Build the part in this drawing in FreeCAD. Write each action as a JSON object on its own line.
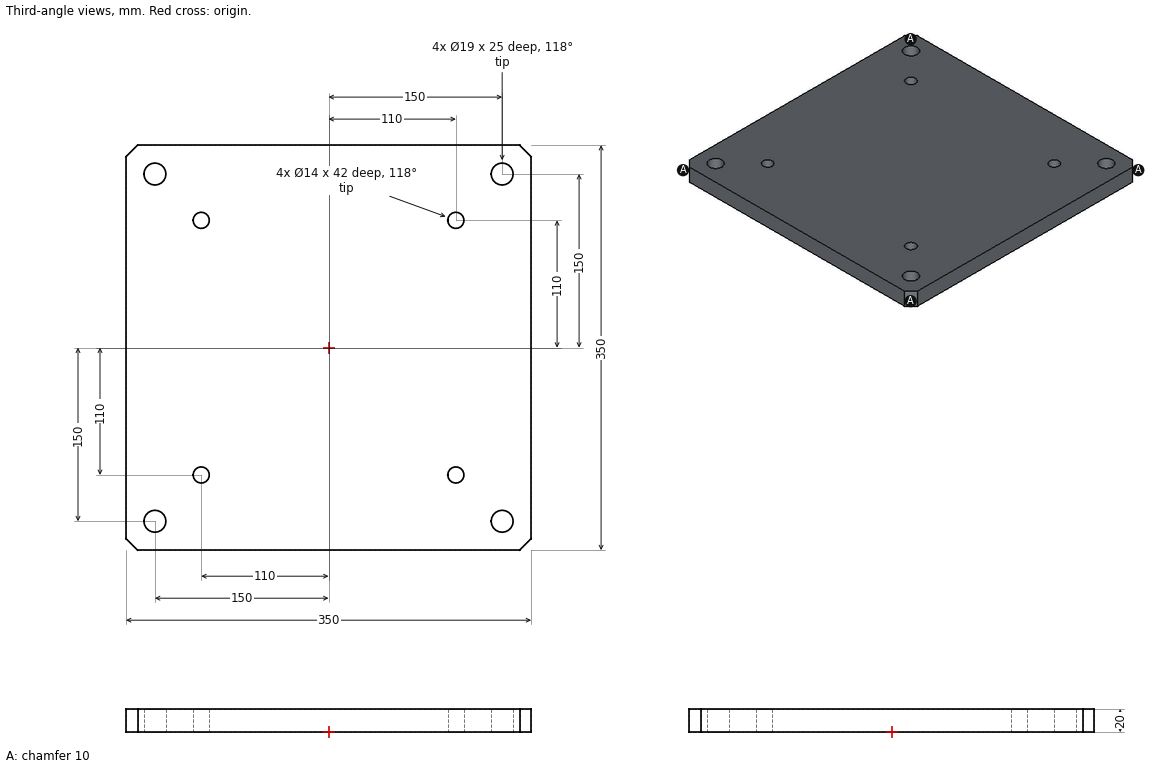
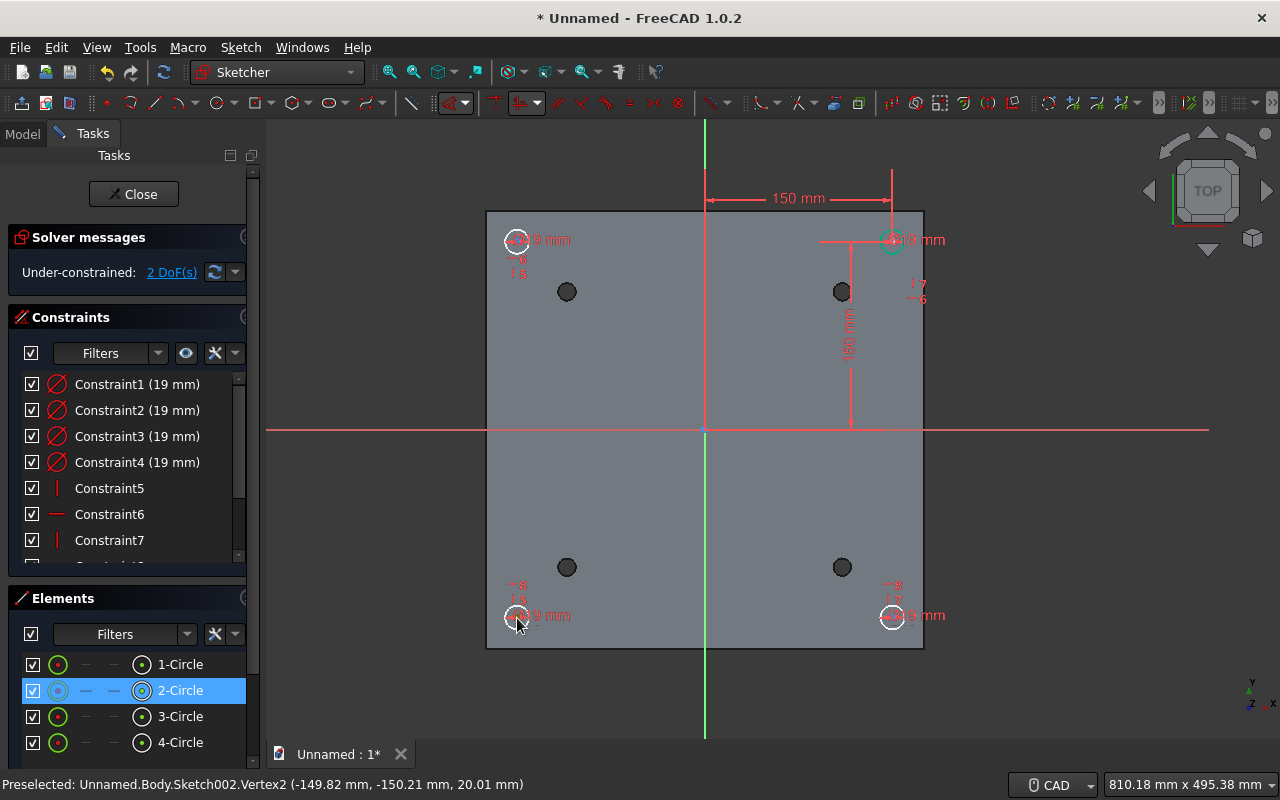
{"action": "key", "text": "l"}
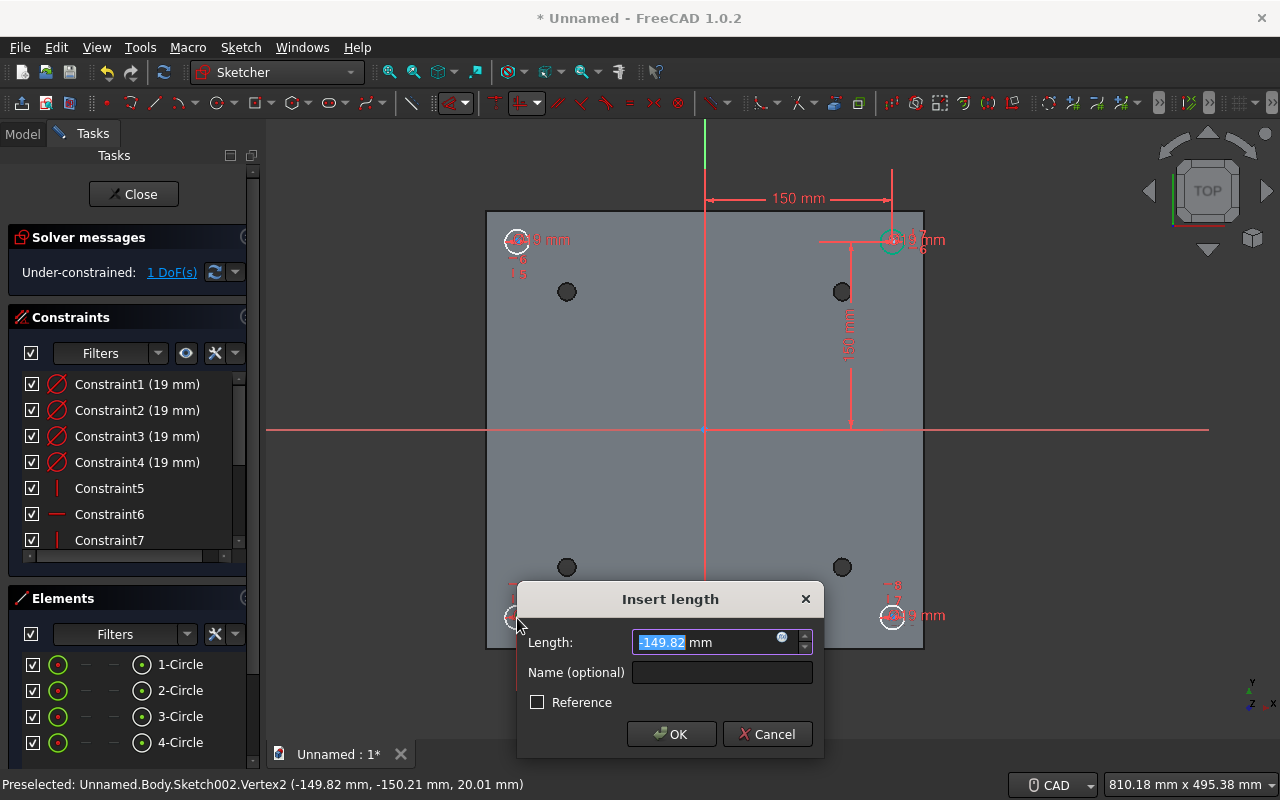
{"action": "type", "text": "-150"}
{"action": "key", "text": "Return"}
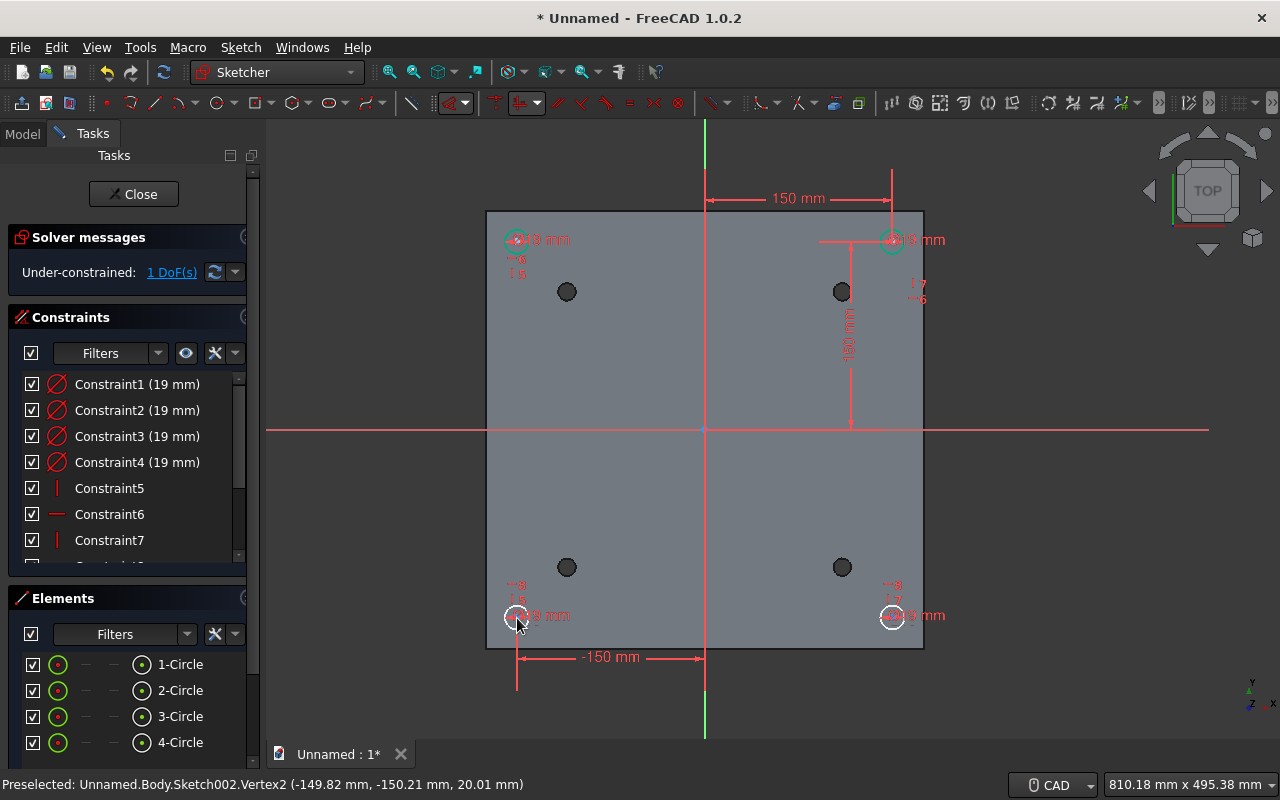
{"action": "left_click", "coordinate": [517, 618]}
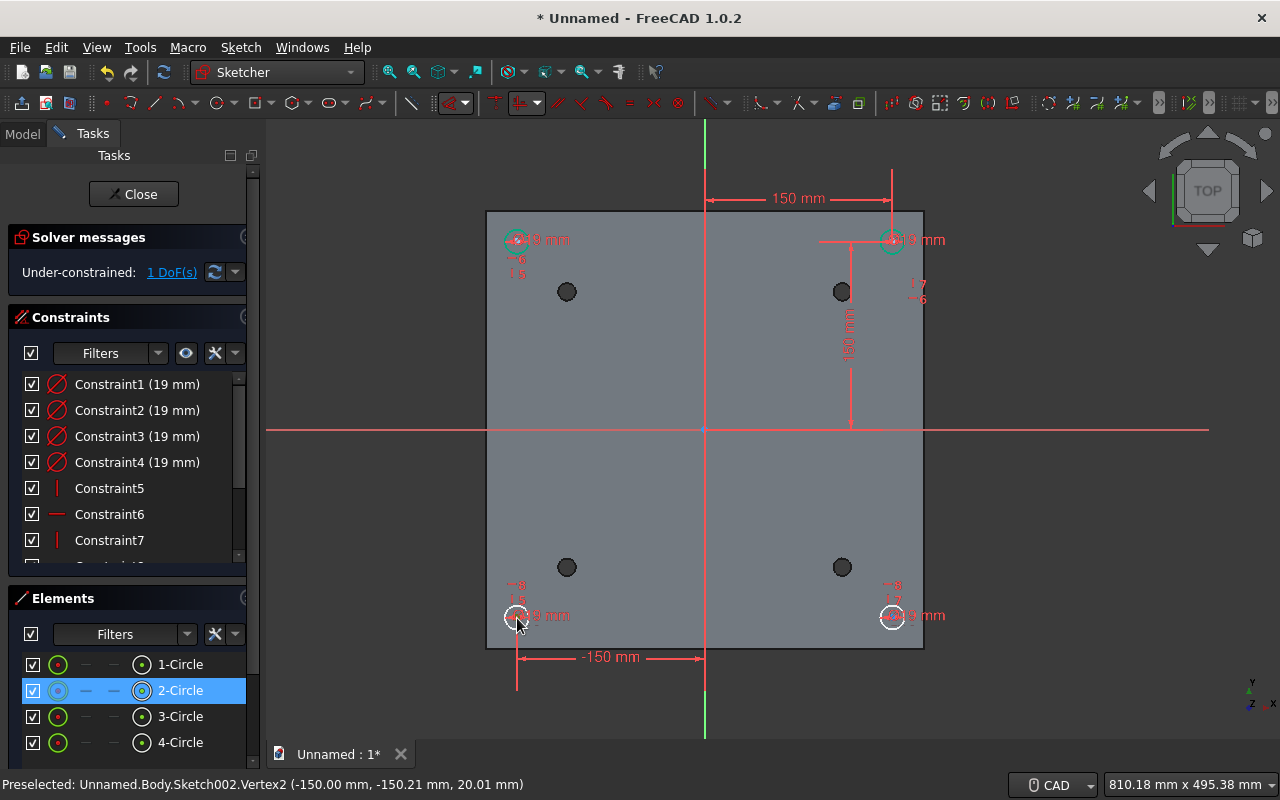
{"action": "key", "text": "i"}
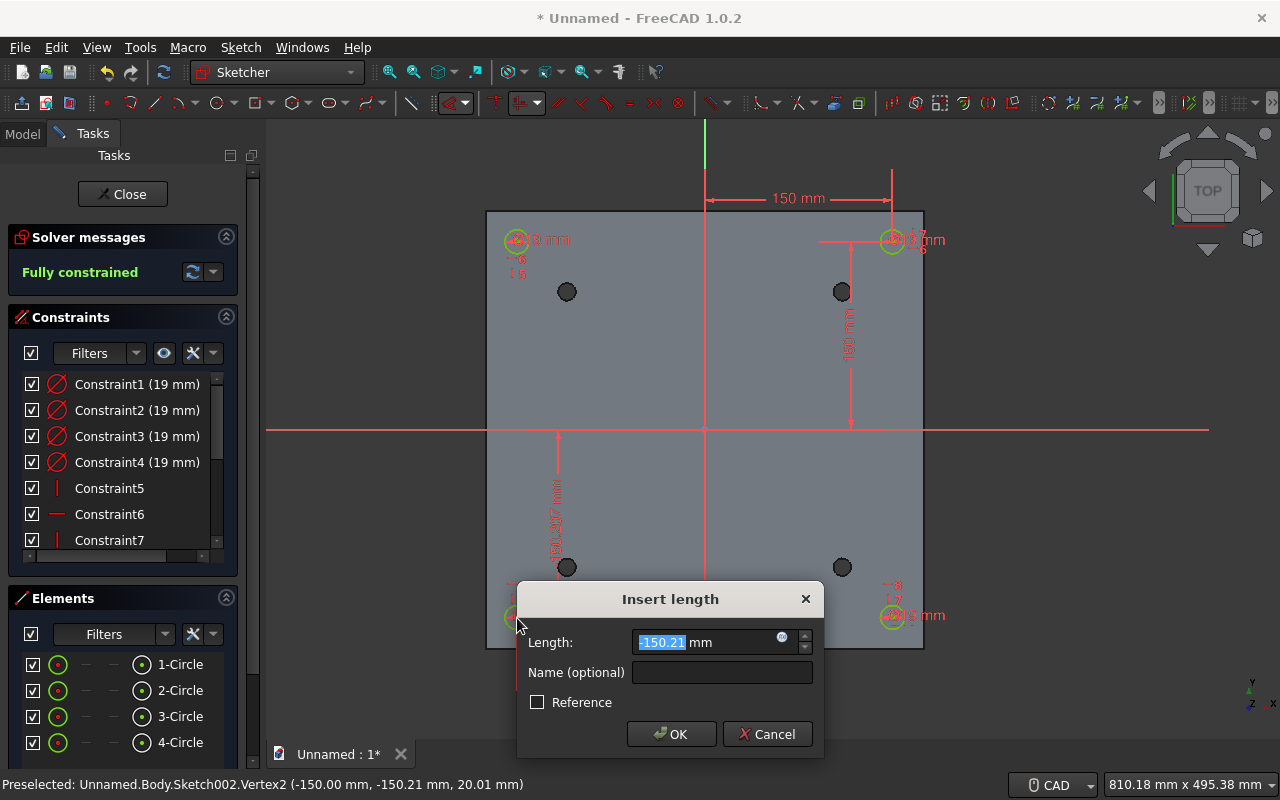
{"action": "type", "text": "-150"}
{"action": "key", "text": "Return"}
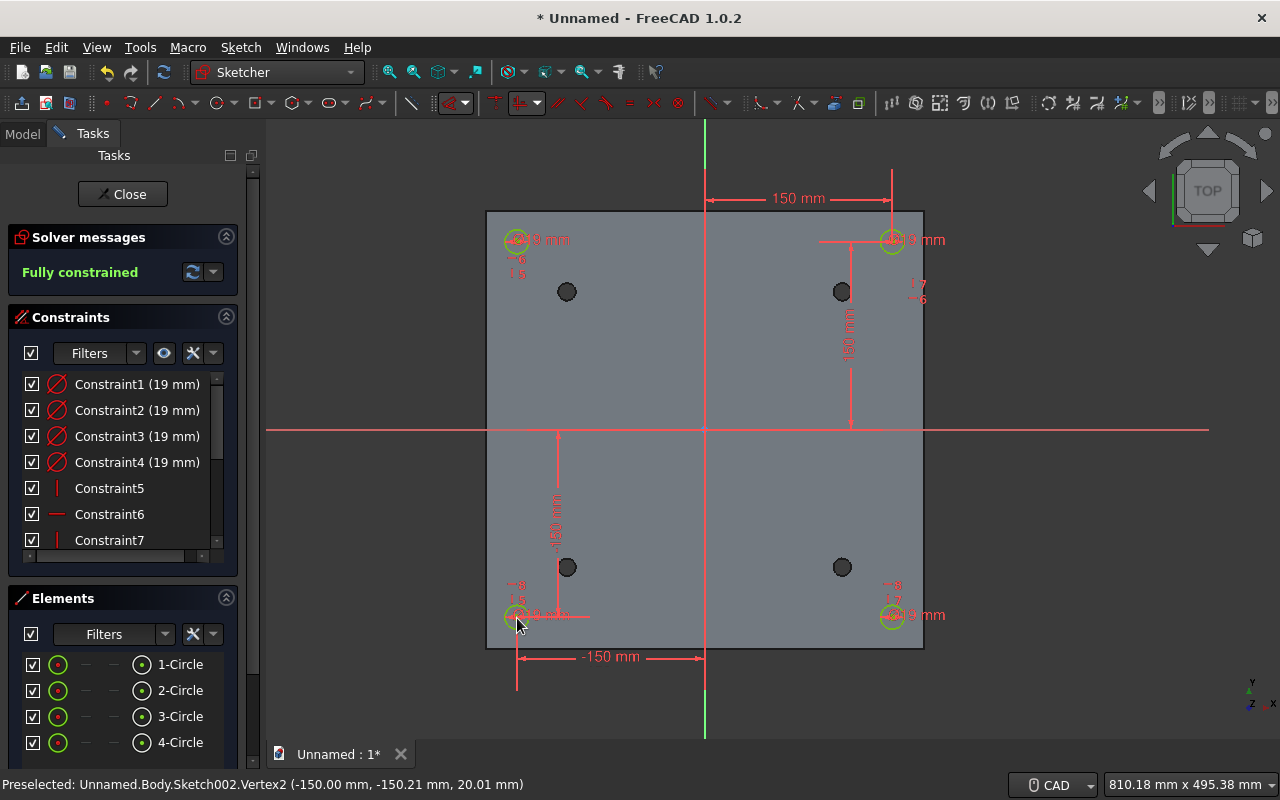
{"action": "left_click", "coordinate": [123, 194]}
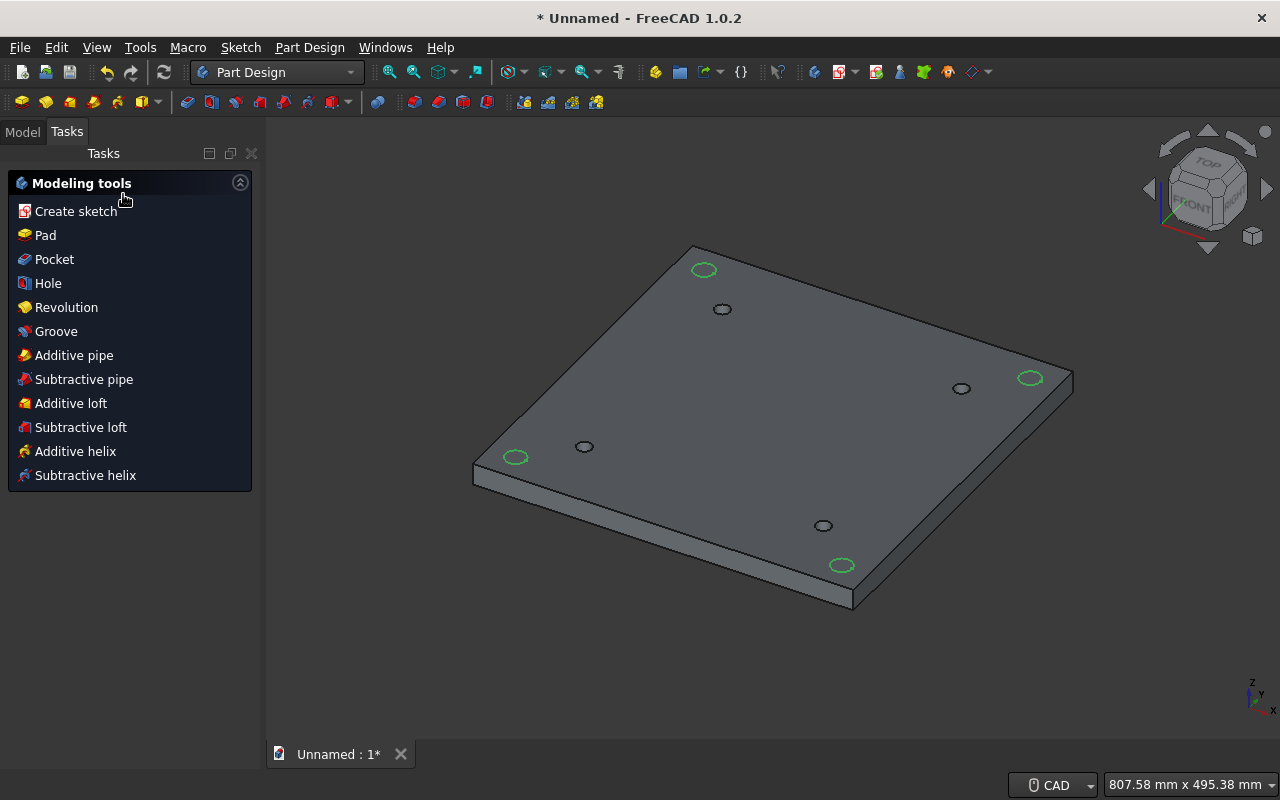
{"action": "left_click", "coordinate": [212, 102]}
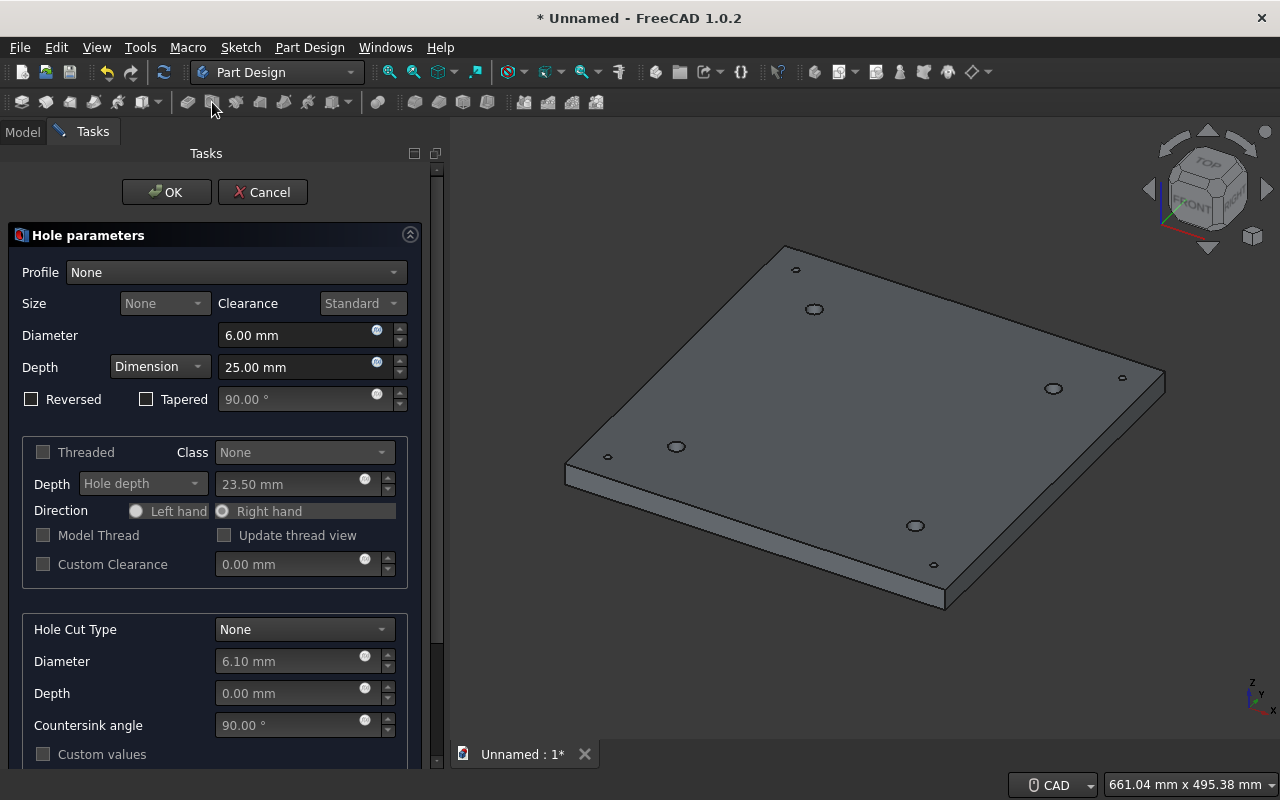
{"action": "triple_click", "coordinate": [305, 335]}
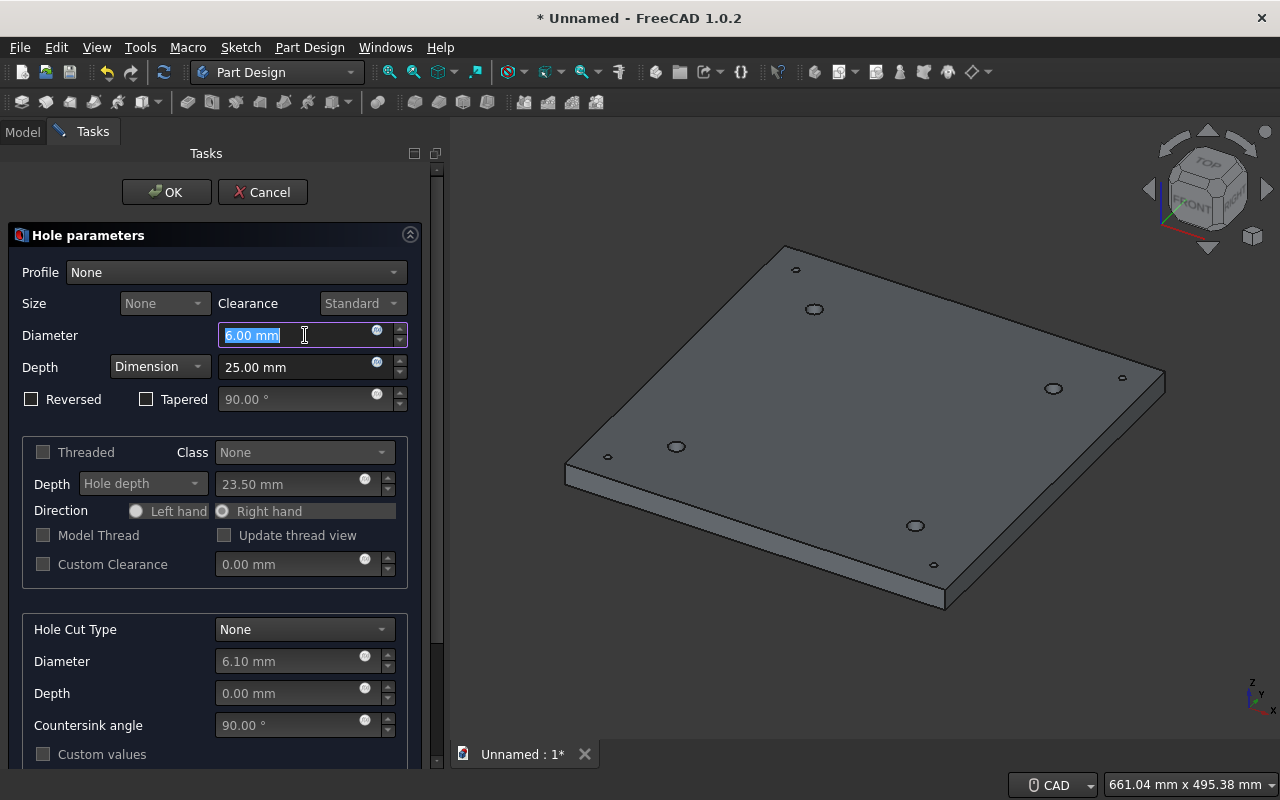
{"action": "type", "text": "19"}
{"action": "key", "text": "Tab"}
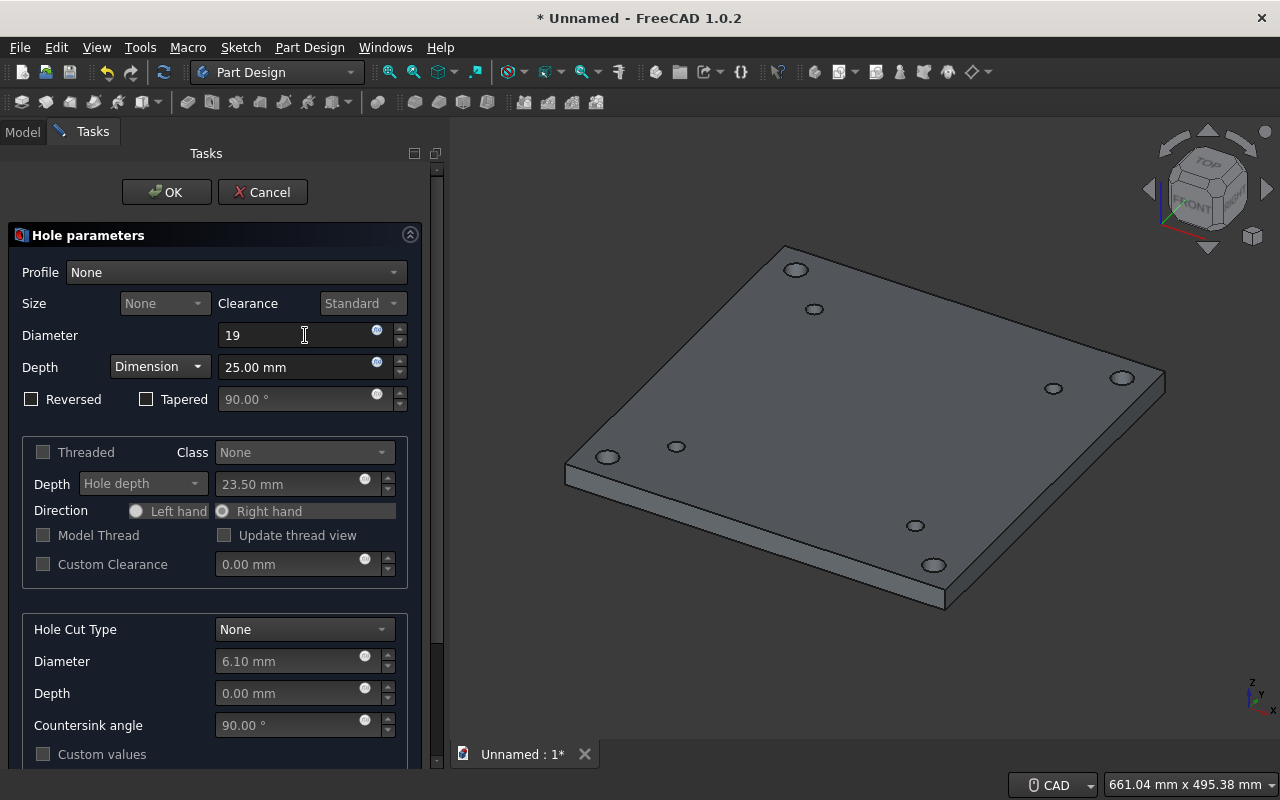
{"action": "triple_click", "coordinate": [305, 367]}